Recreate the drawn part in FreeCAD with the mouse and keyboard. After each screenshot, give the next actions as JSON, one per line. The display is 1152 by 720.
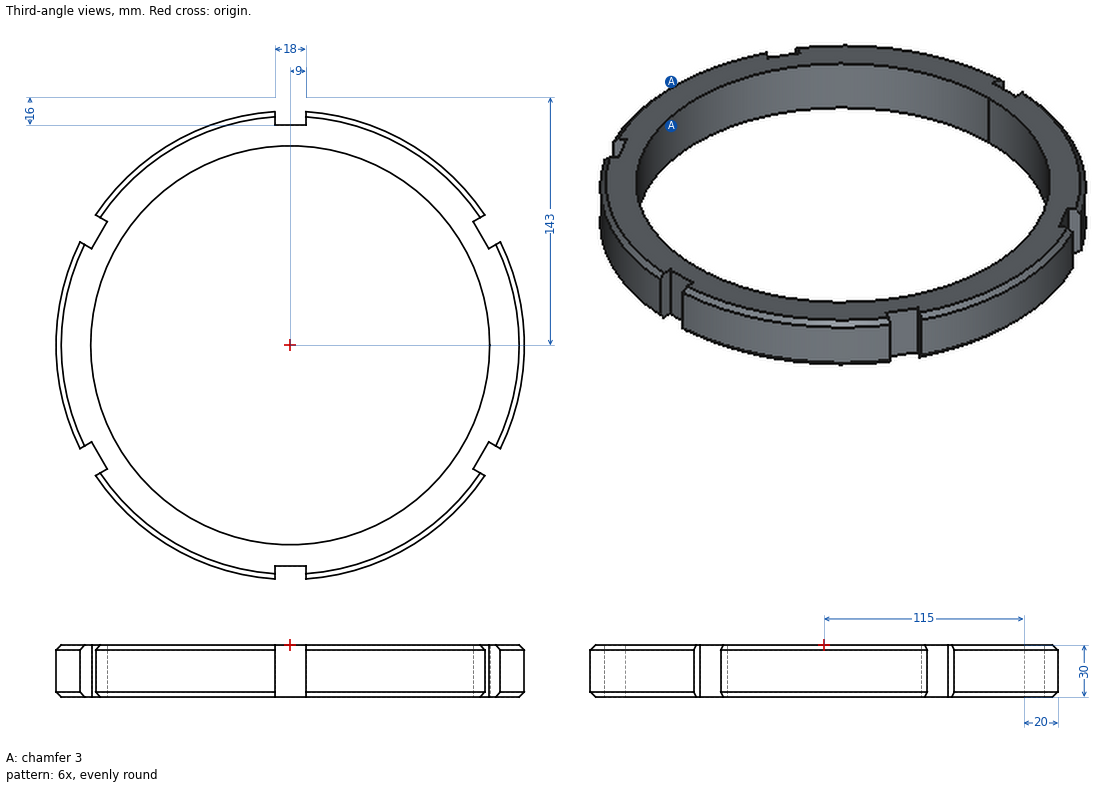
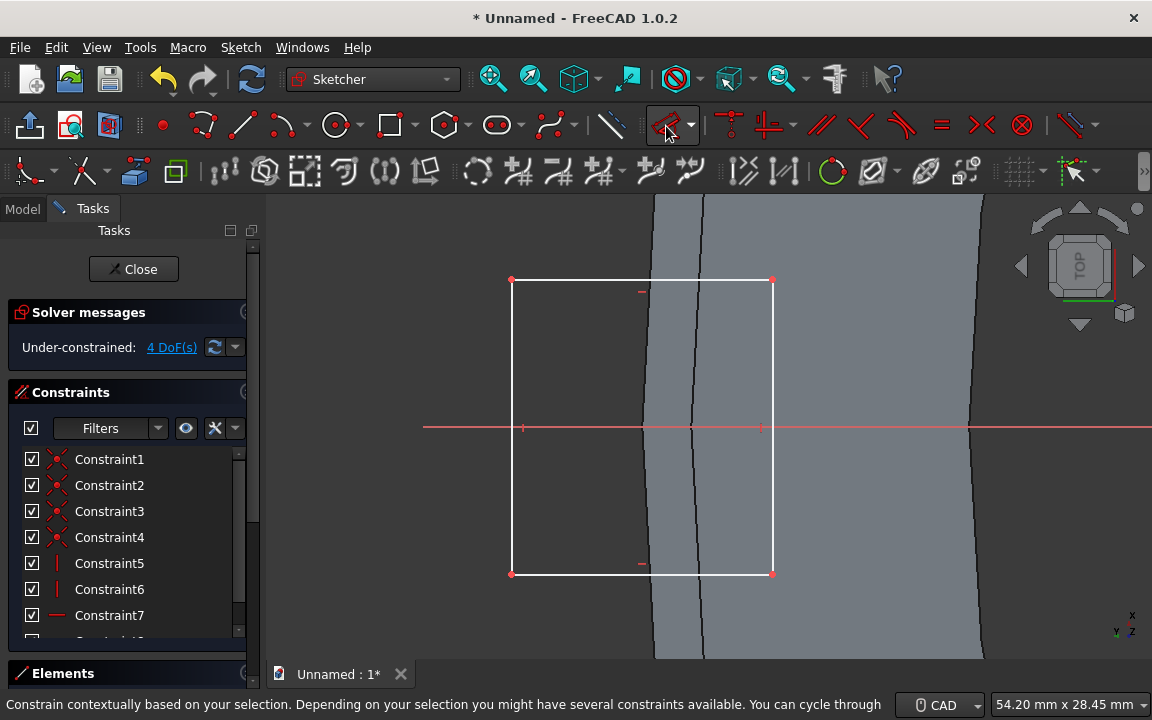
{"action": "left_click", "coordinate": [512, 369]}
{"action": "left_click", "coordinate": [478, 360]}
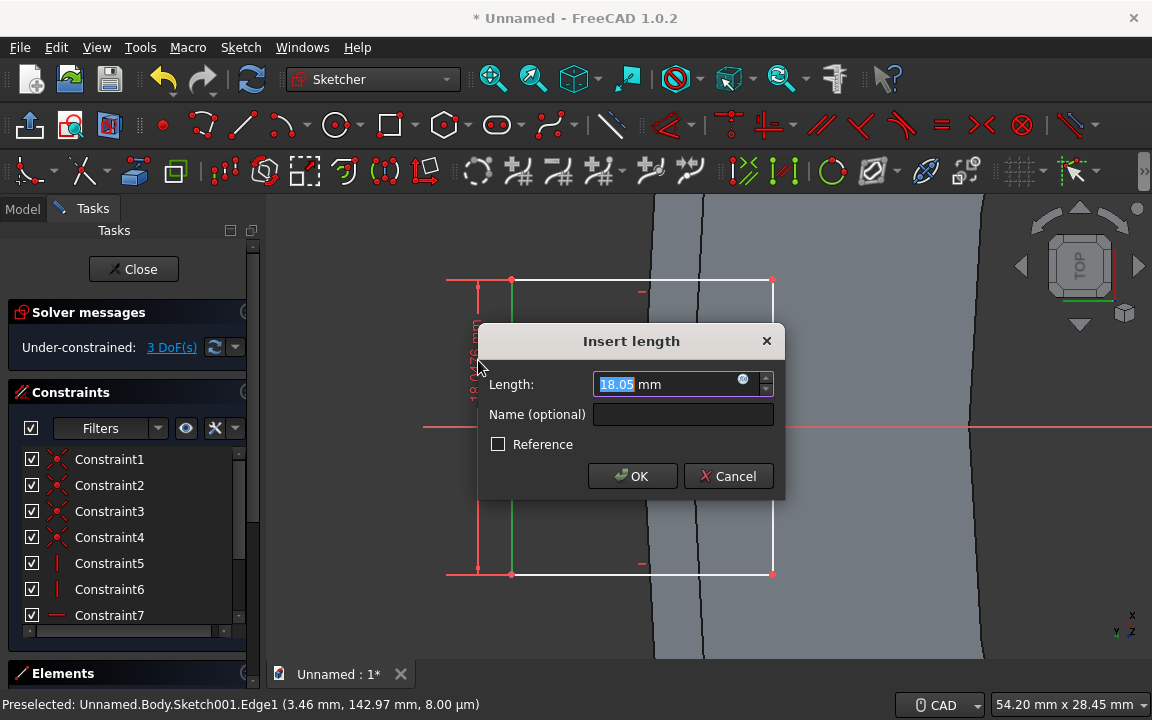
{"action": "type", "text": "18"}
{"action": "key", "text": "Return"}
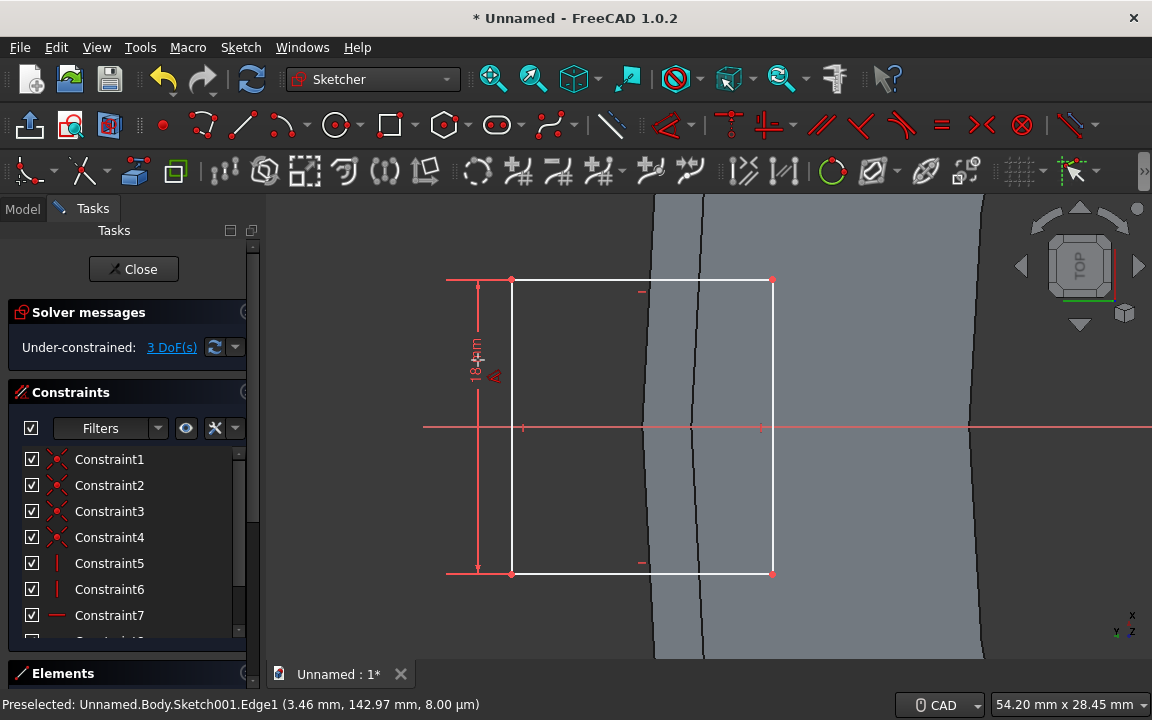
{"action": "left_click", "coordinate": [590, 574]}
{"action": "left_click", "coordinate": [642, 608]}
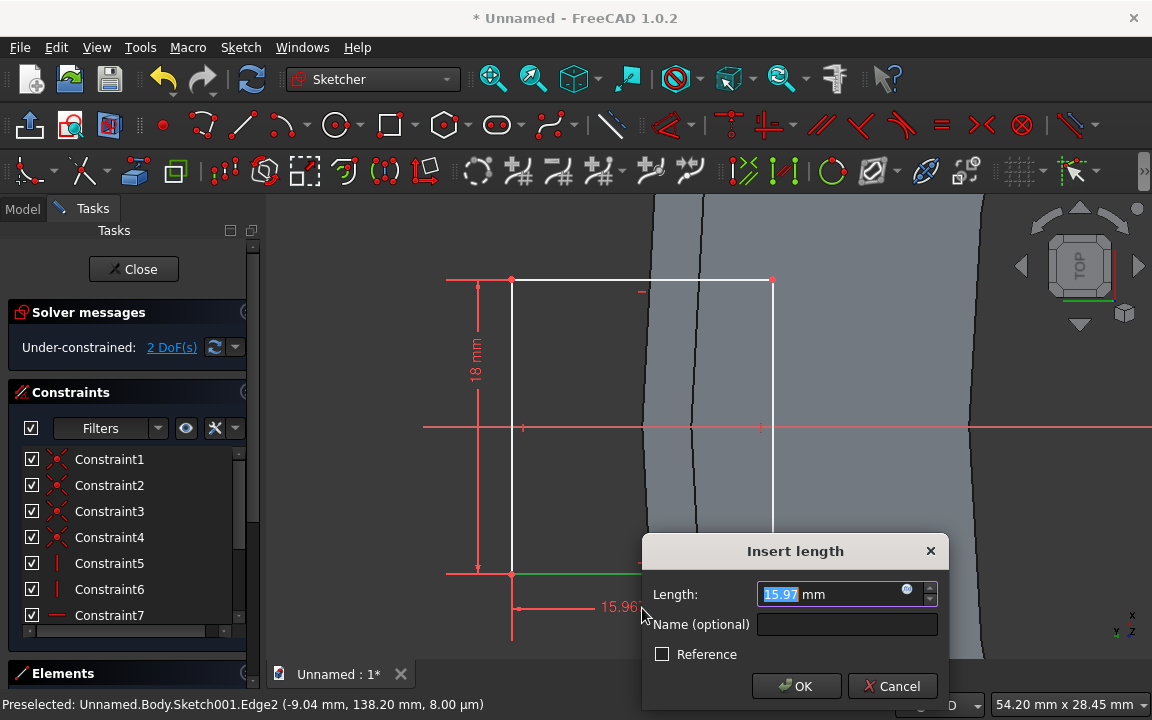
{"action": "type", "text": "16"}
{"action": "key", "text": "Return"}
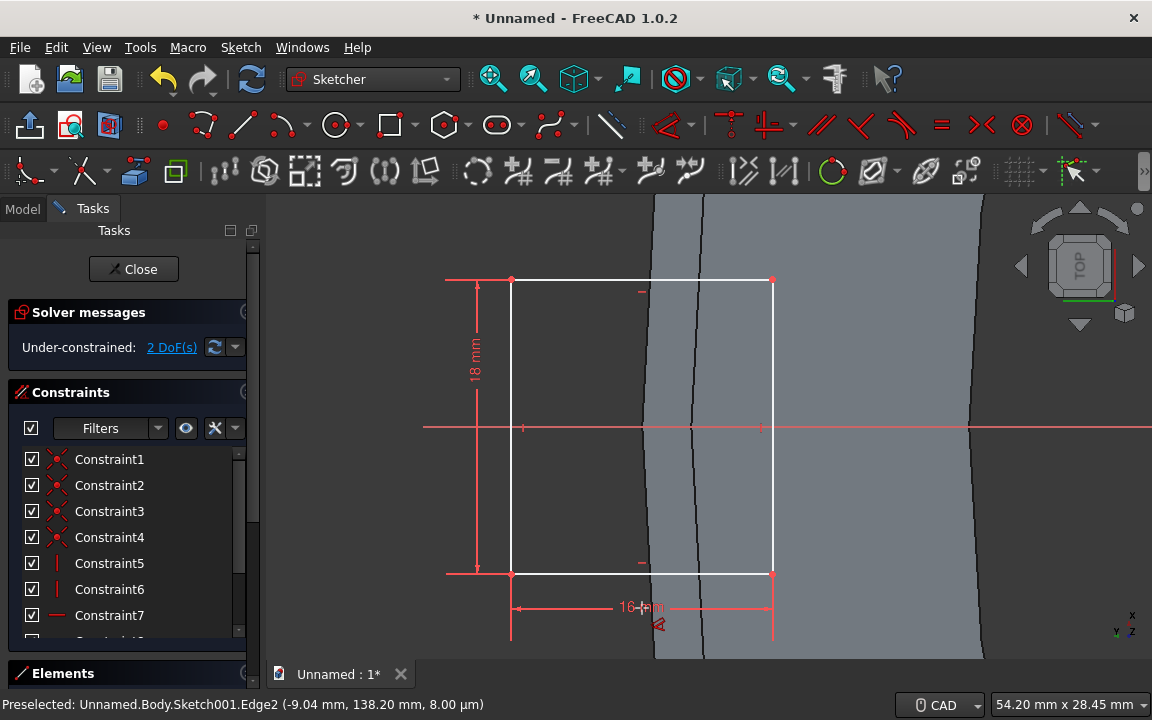
{"action": "left_click", "coordinate": [511, 280]}
{"action": "left_click", "coordinate": [477, 320]}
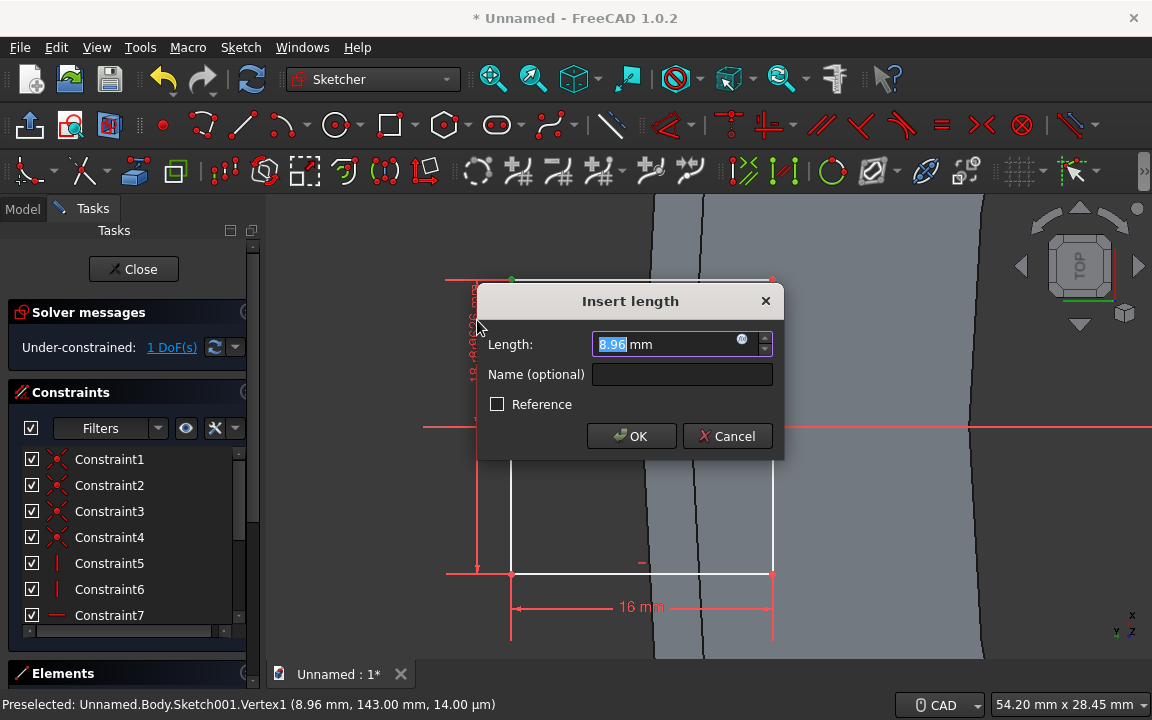
{"action": "type", "text": "9"}
{"action": "key", "text": "Return"}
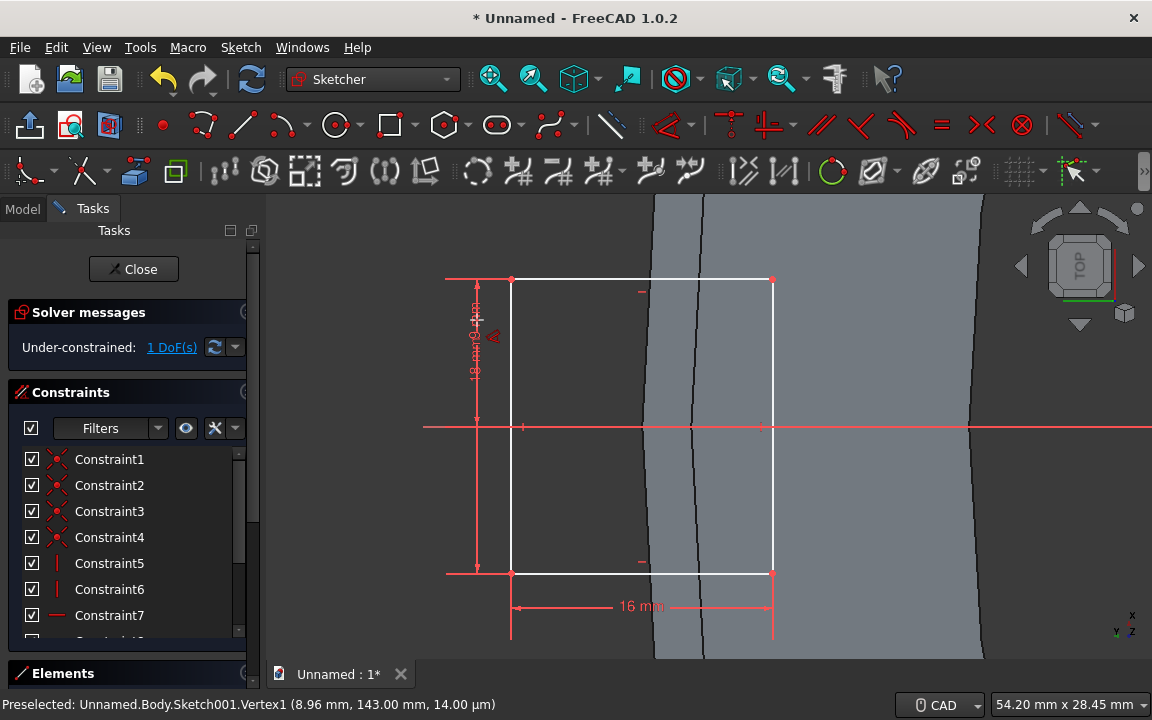
{"action": "left_click", "coordinate": [511, 279]}
{"action": "left_click", "coordinate": [749, 245]}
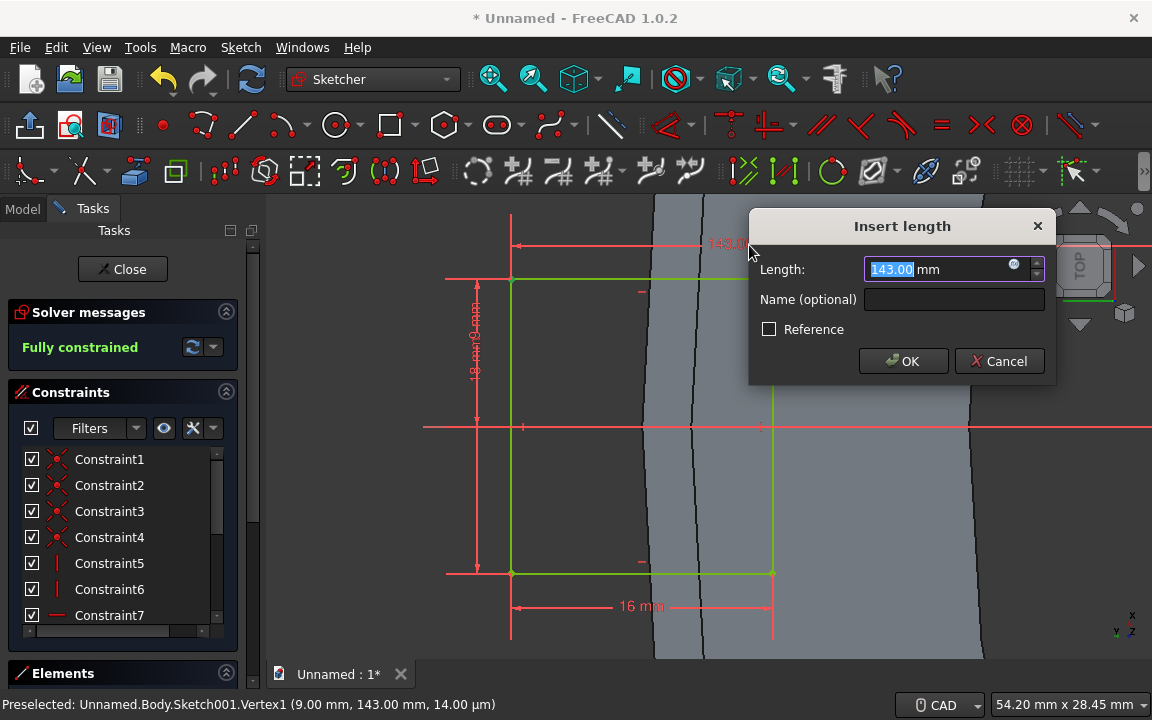
{"action": "type", "text": "143"}
{"action": "key", "text": "Return"}
{"action": "key", "text": "Escape"}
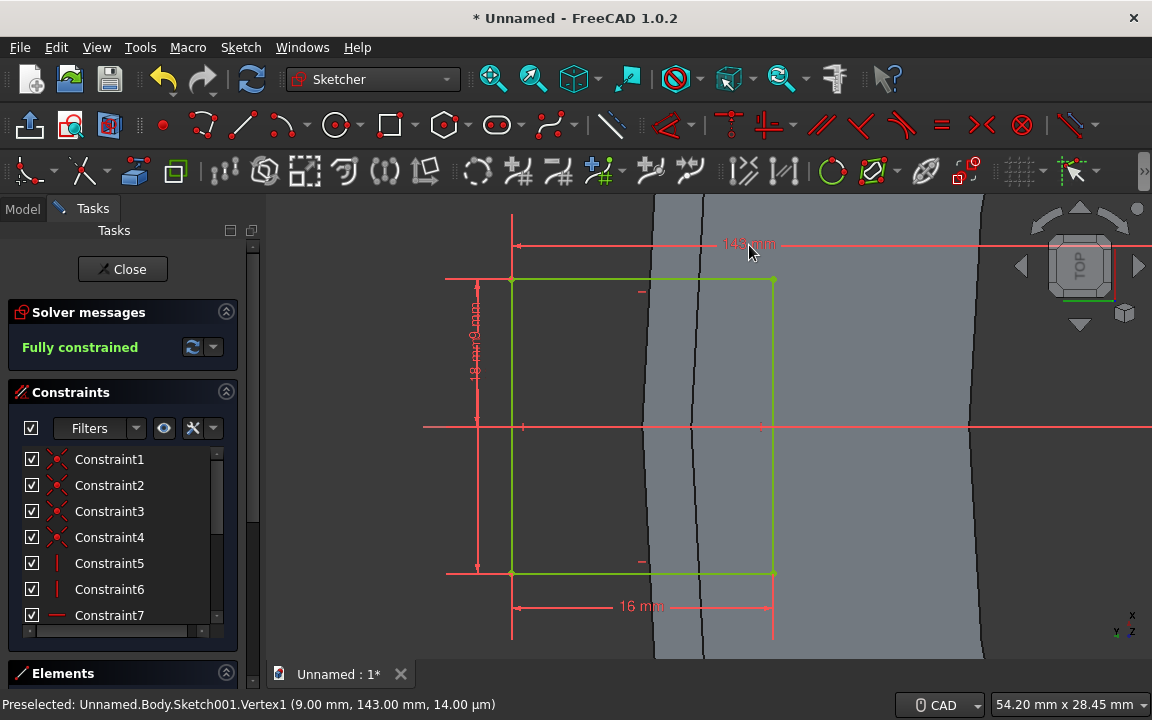
{"action": "left_click", "coordinate": [123, 269]}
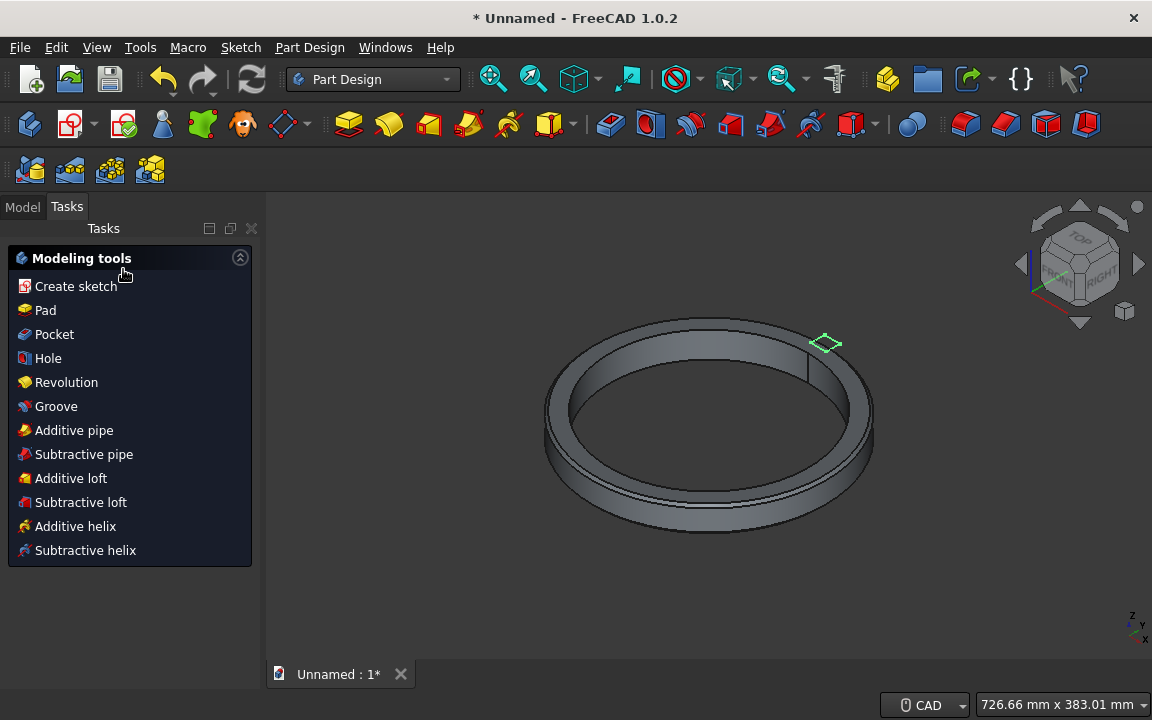
{"action": "left_click", "coordinate": [612, 124]}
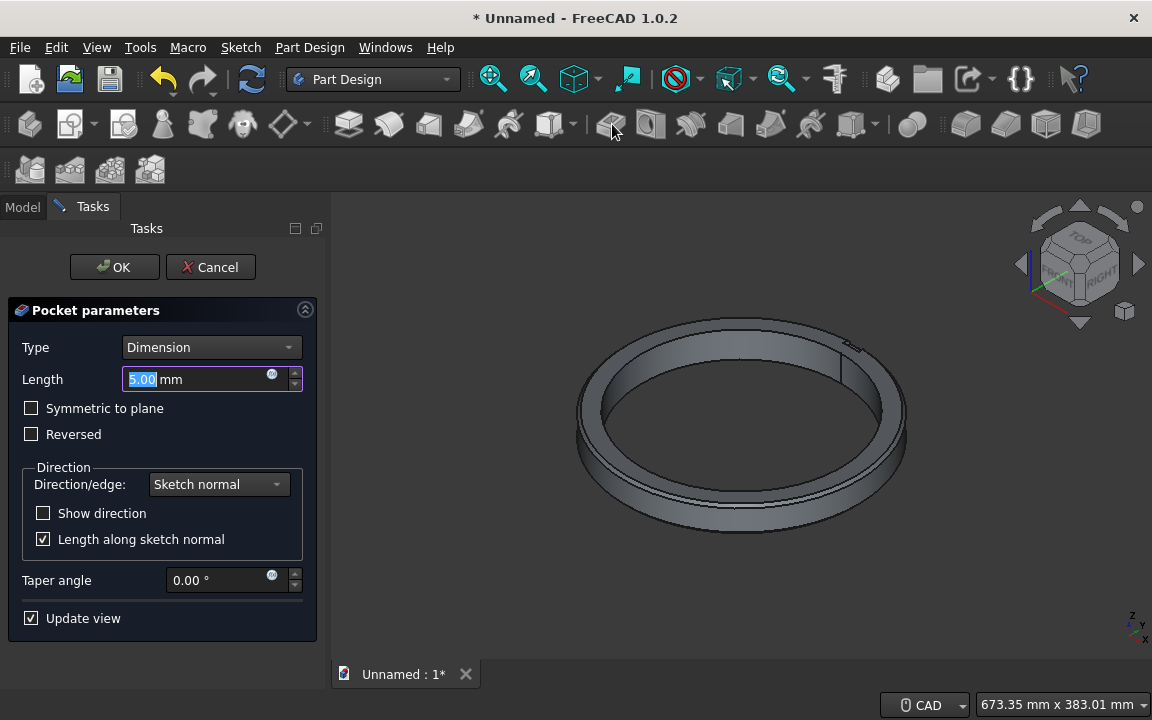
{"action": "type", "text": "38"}
{"action": "key", "text": "Tab"}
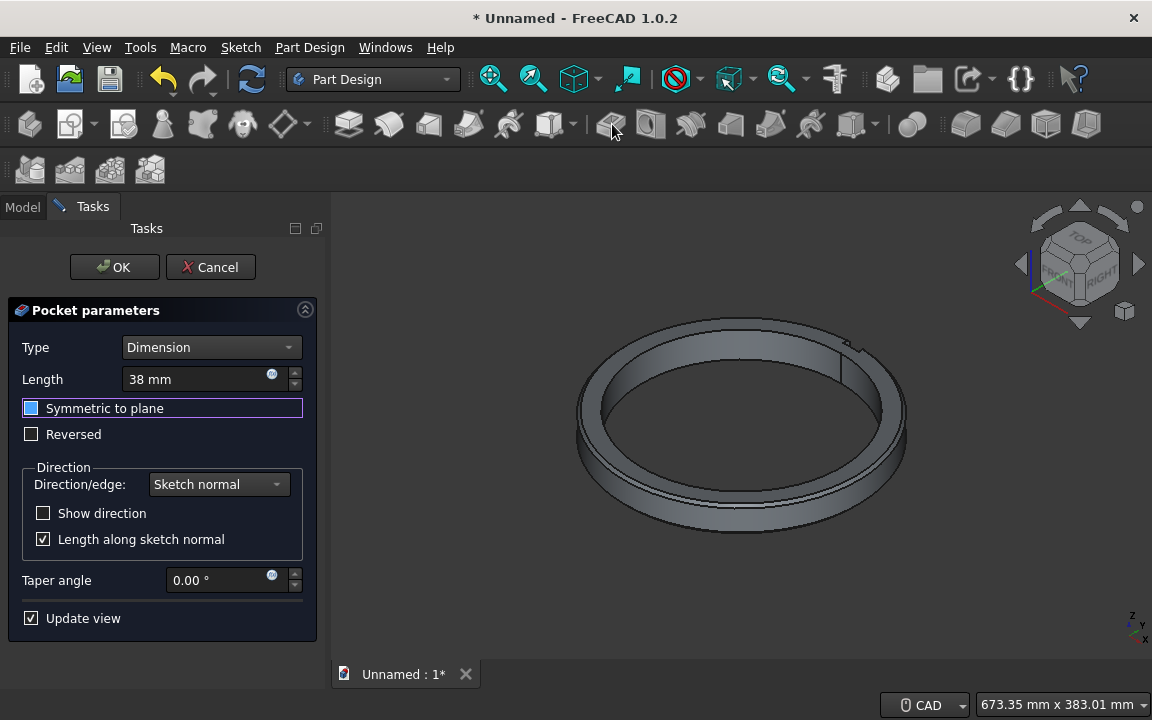
{"action": "left_click", "coordinate": [115, 267]}